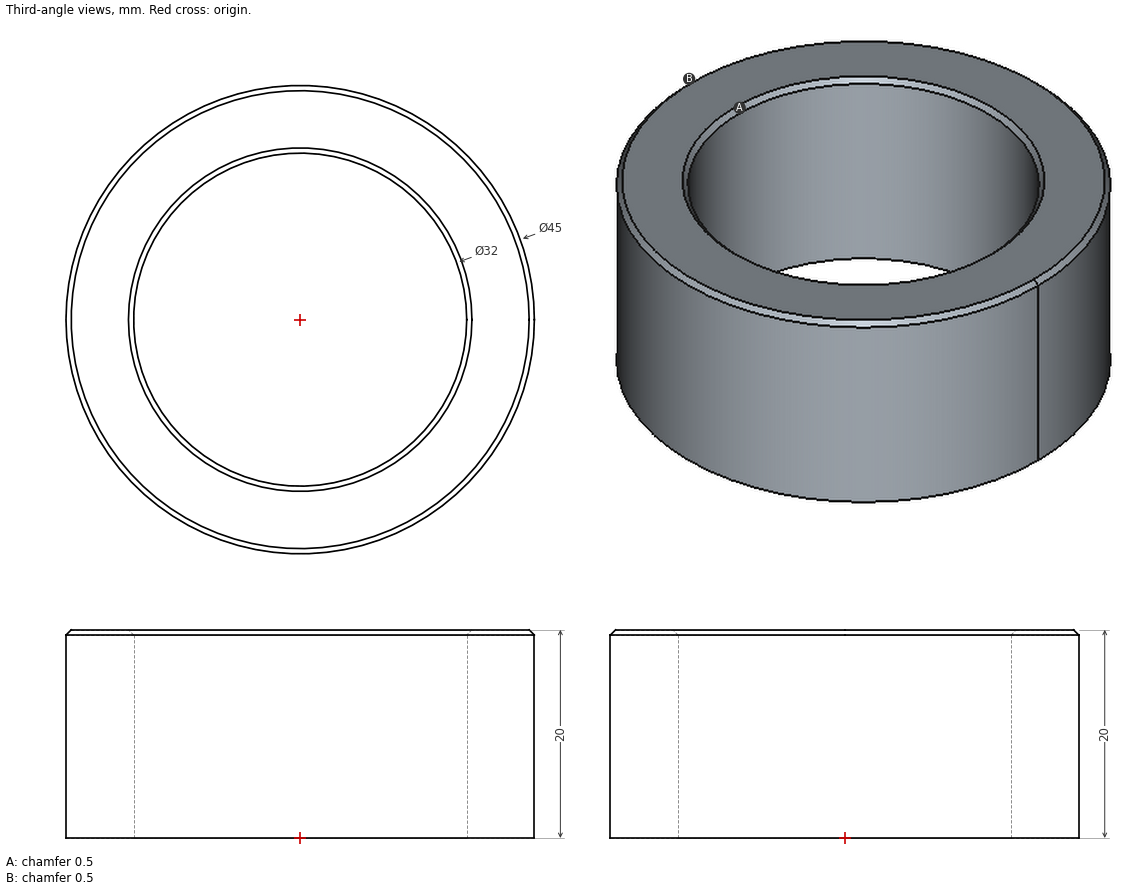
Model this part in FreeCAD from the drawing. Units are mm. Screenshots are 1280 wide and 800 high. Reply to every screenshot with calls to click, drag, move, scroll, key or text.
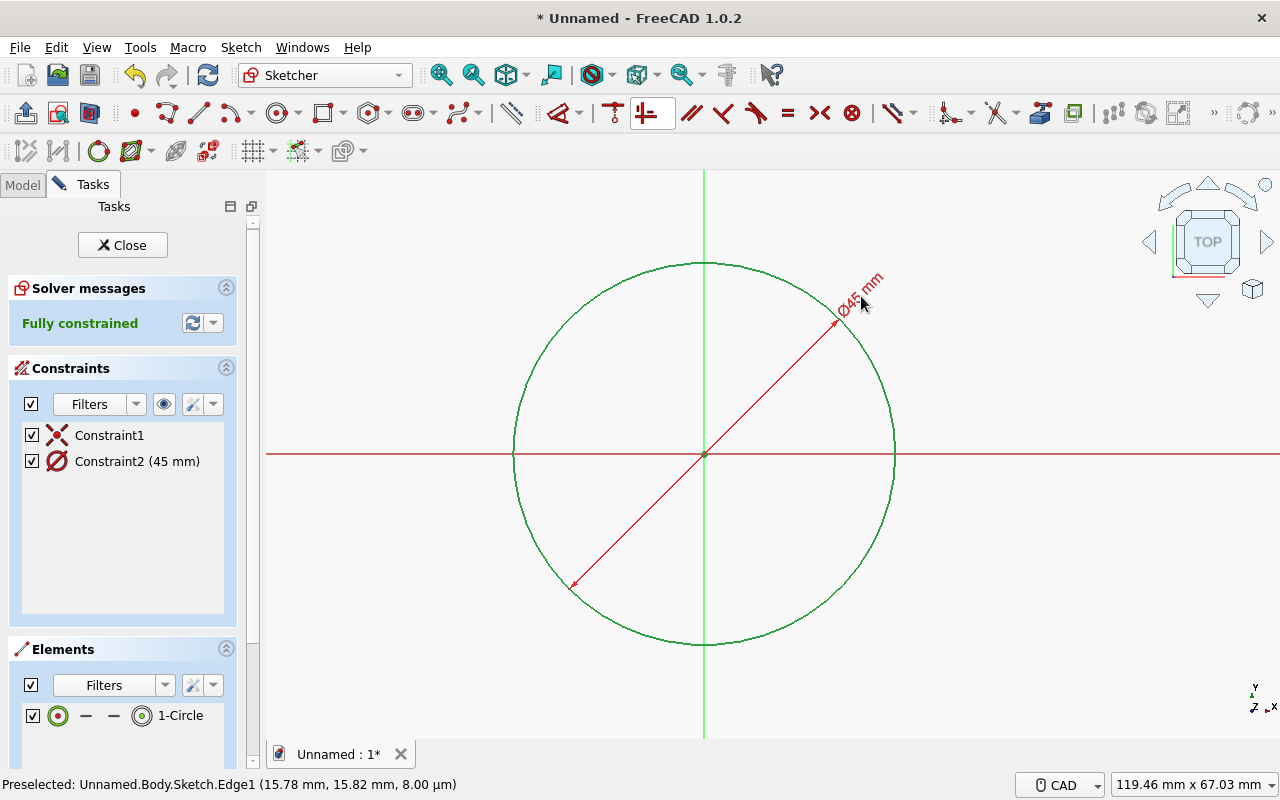
click(123, 245)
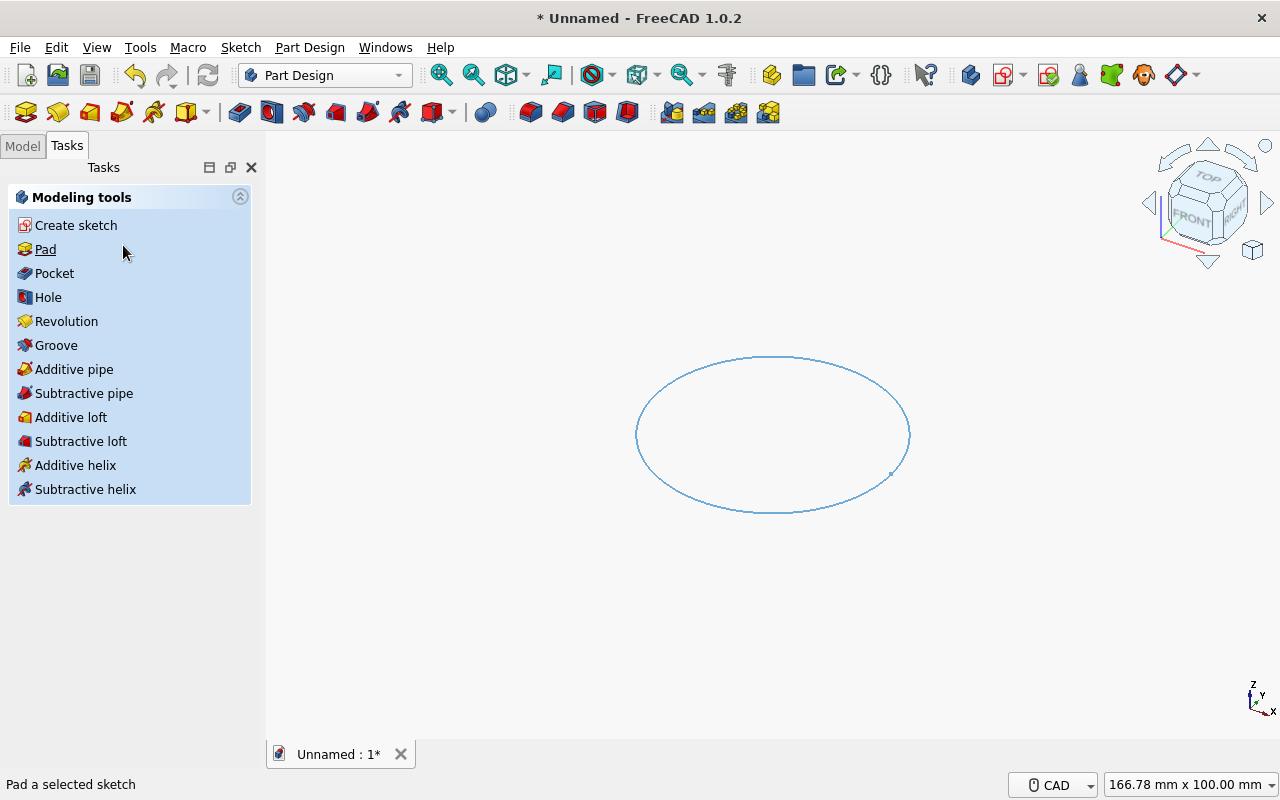
click(26, 112)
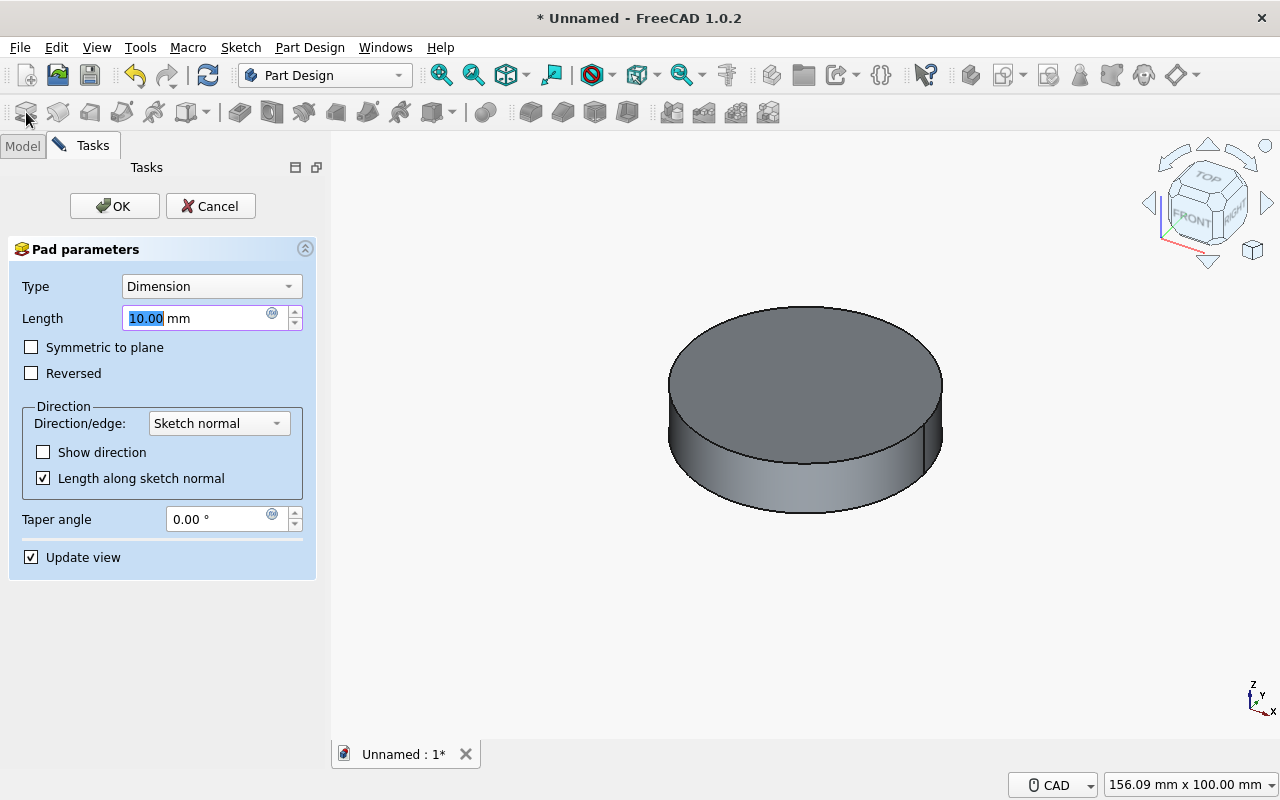
text(20)
key(Tab)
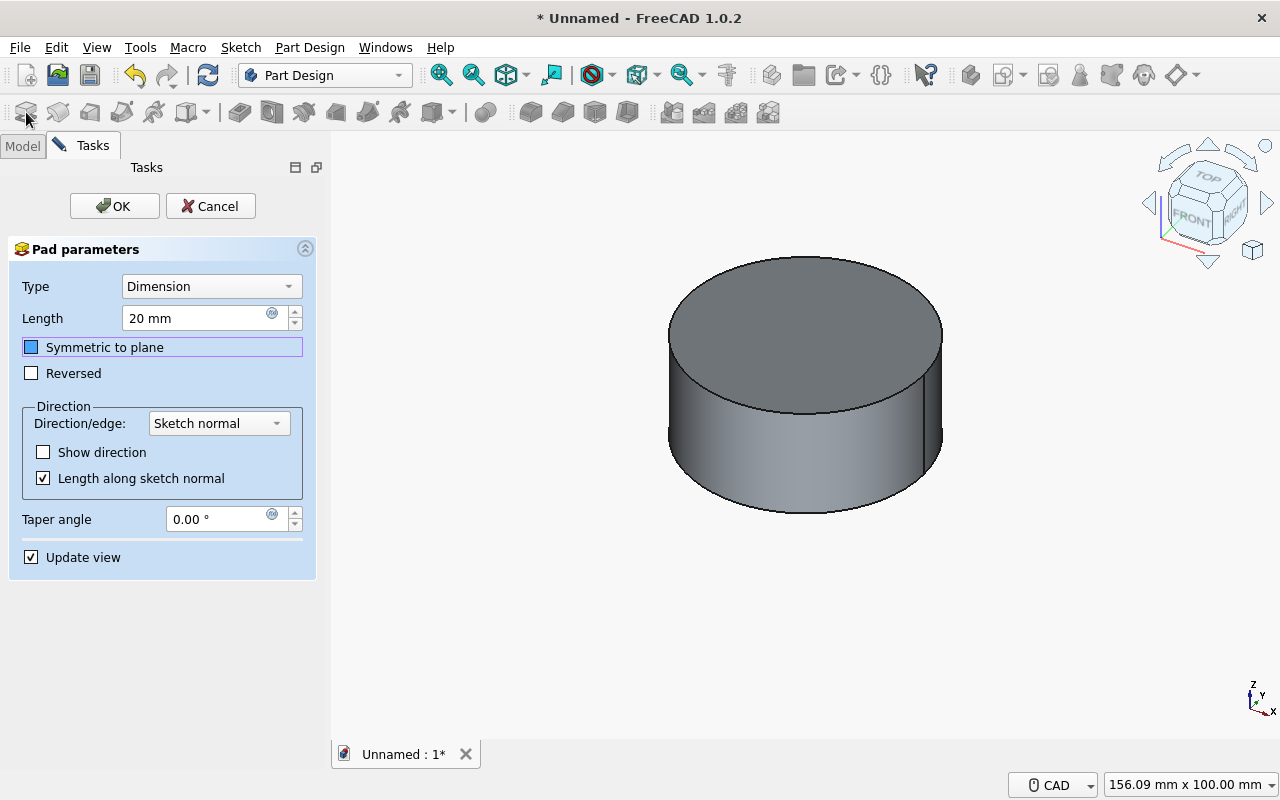
click(115, 206)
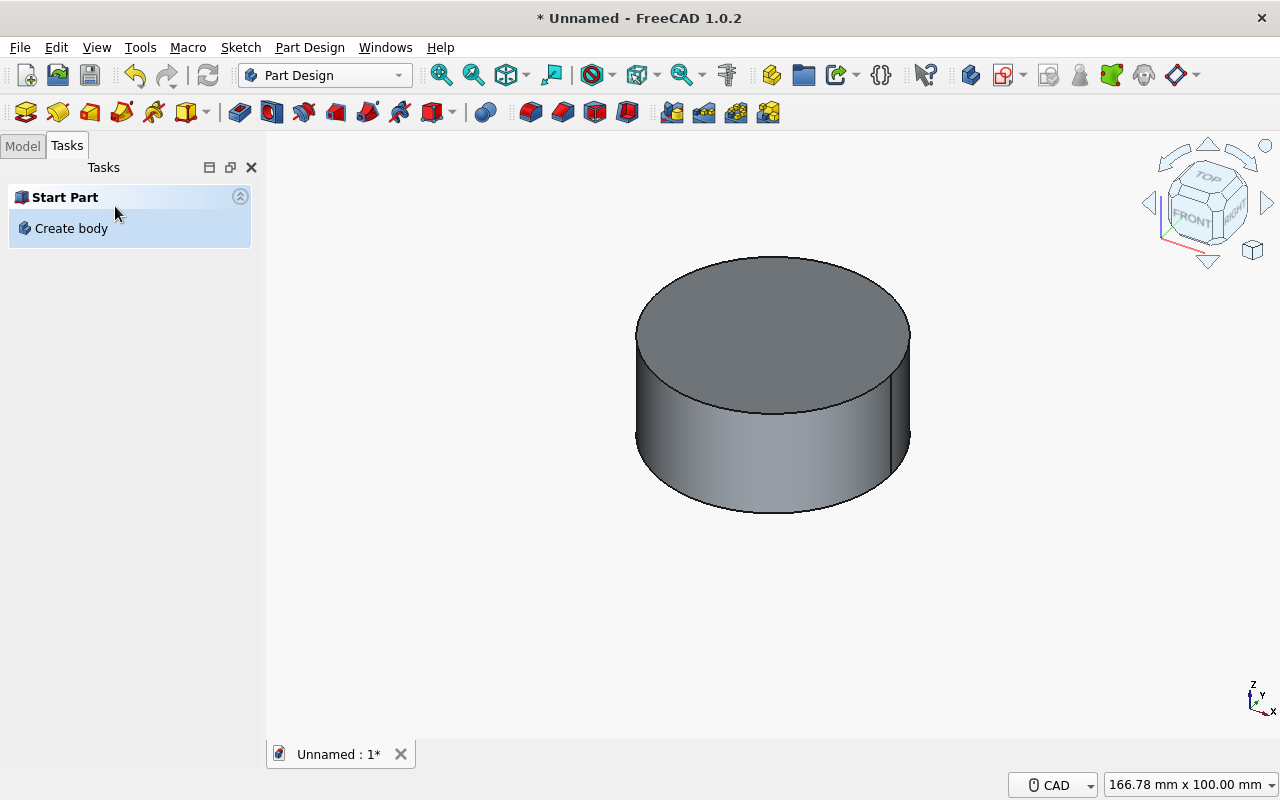
click(773, 334)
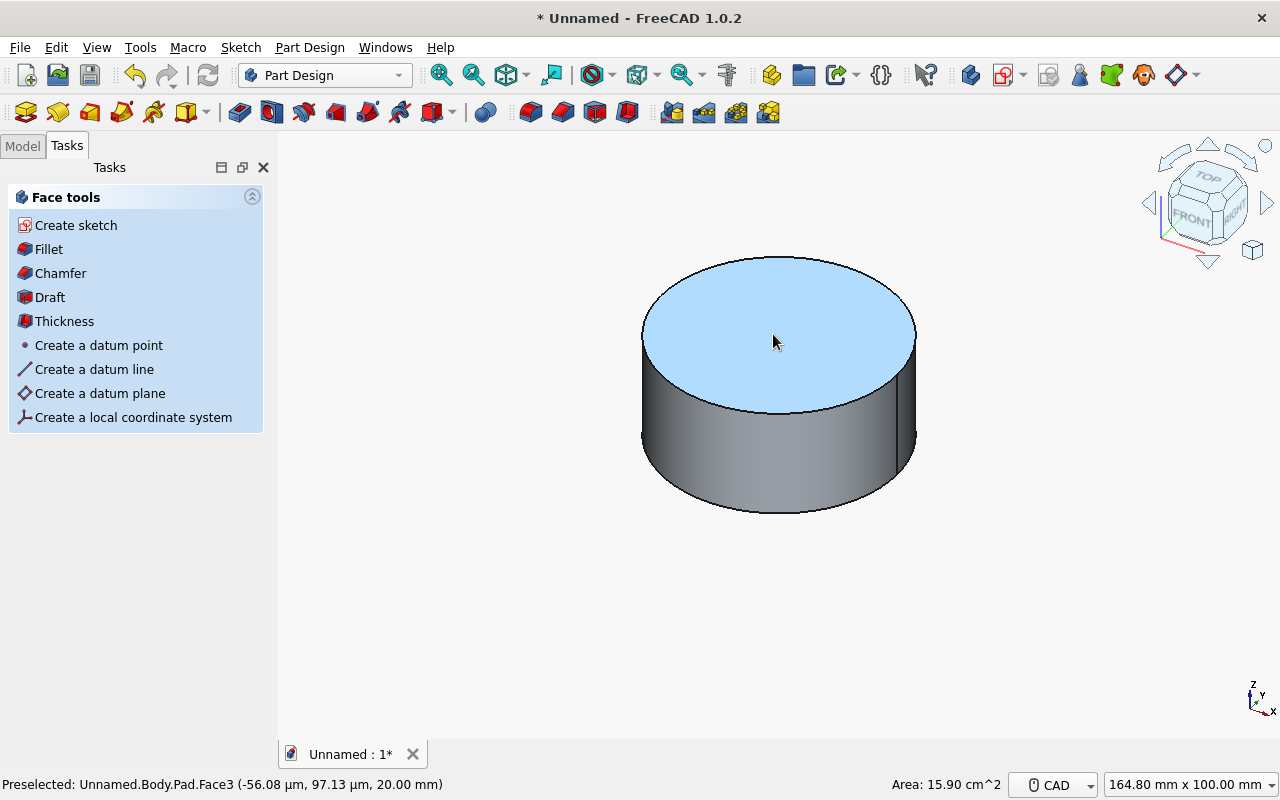
click(1004, 76)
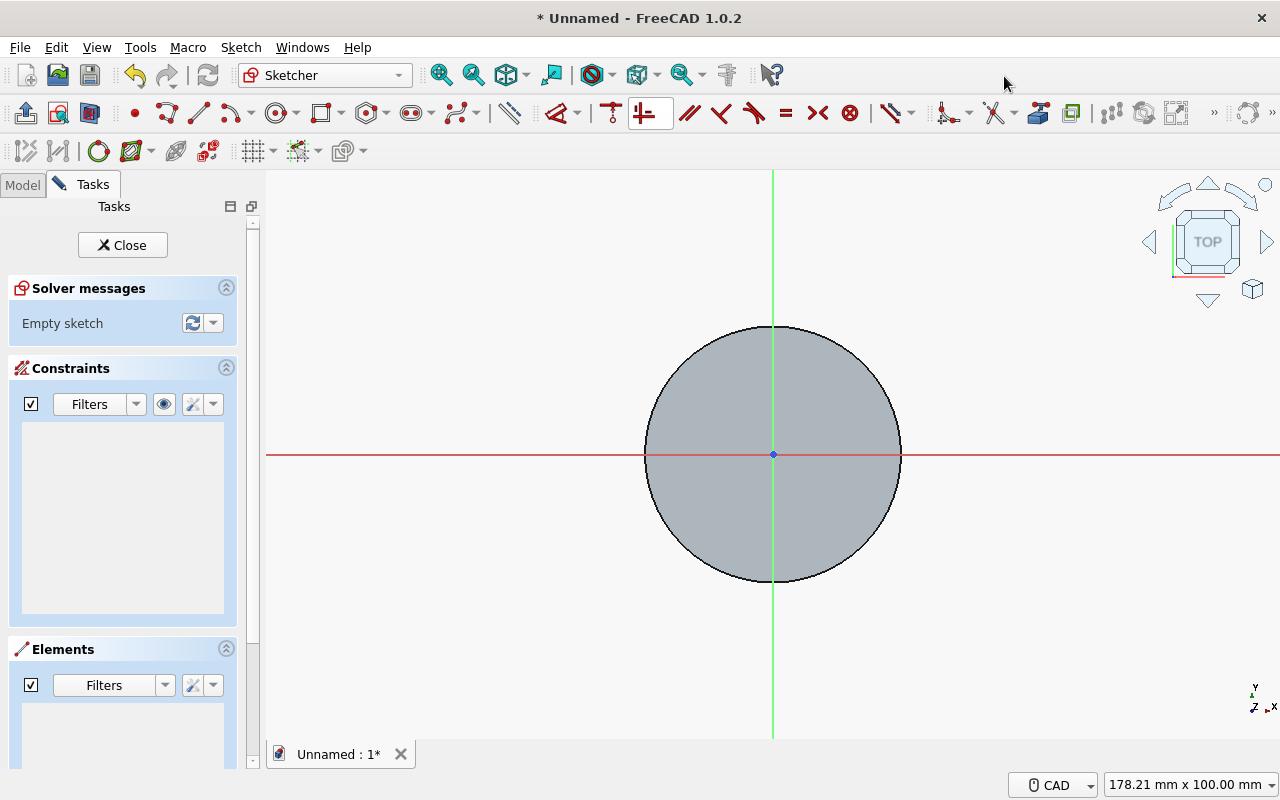
scroll(856, 454, up, 3)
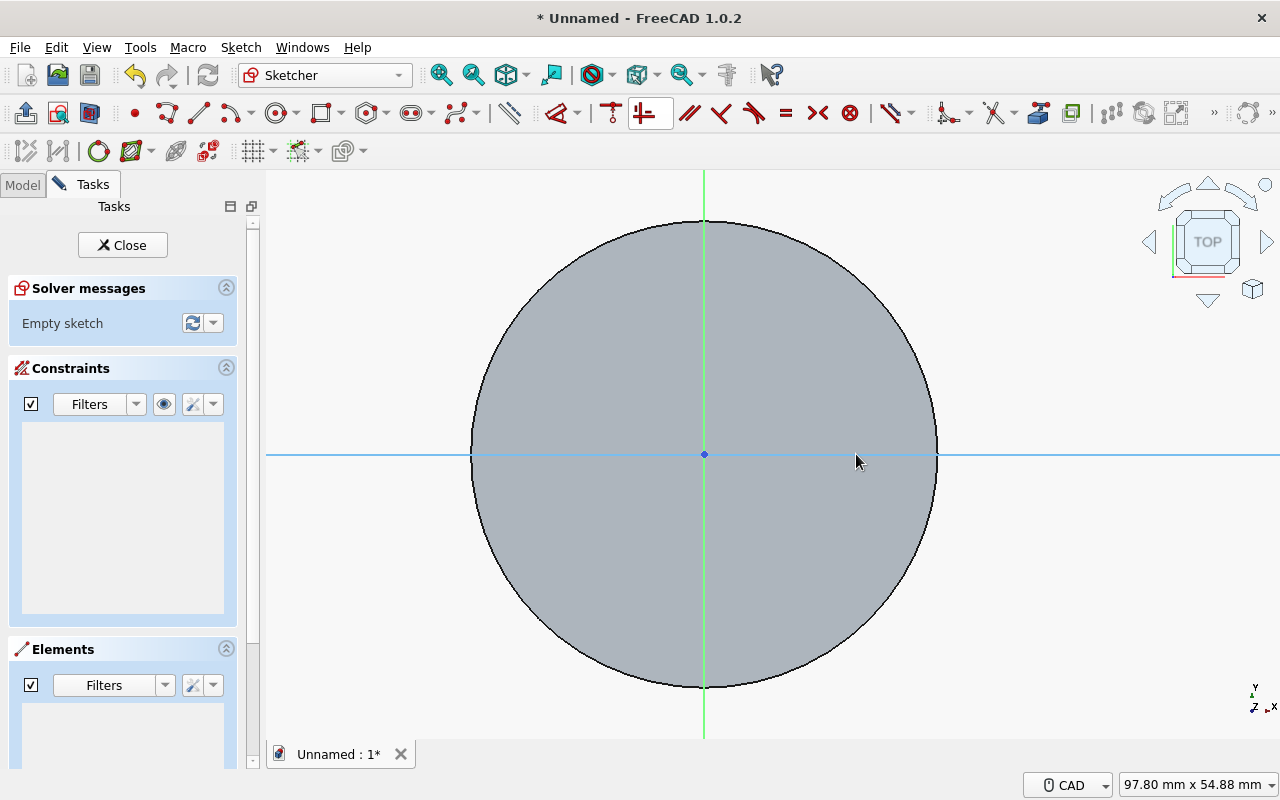
key(g)
key(c)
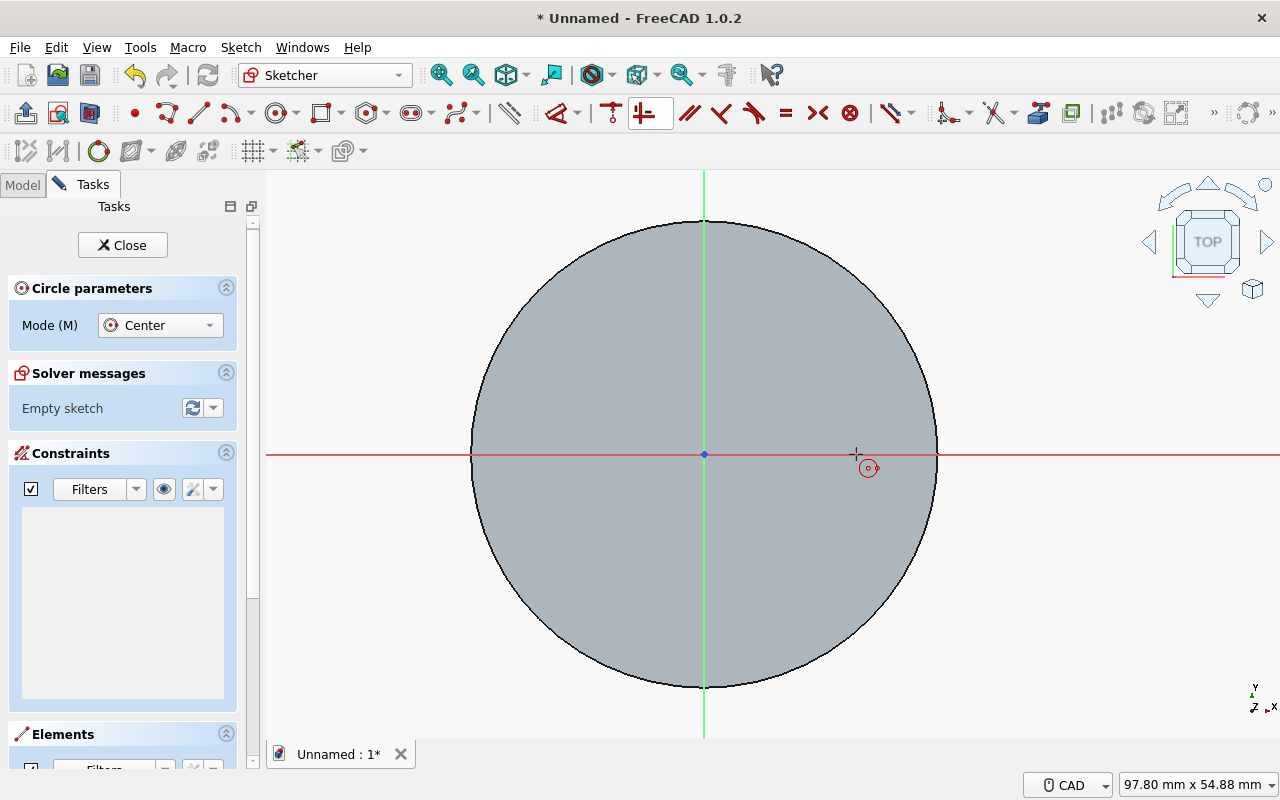
click(704, 454)
click(822, 337)
key(Escape)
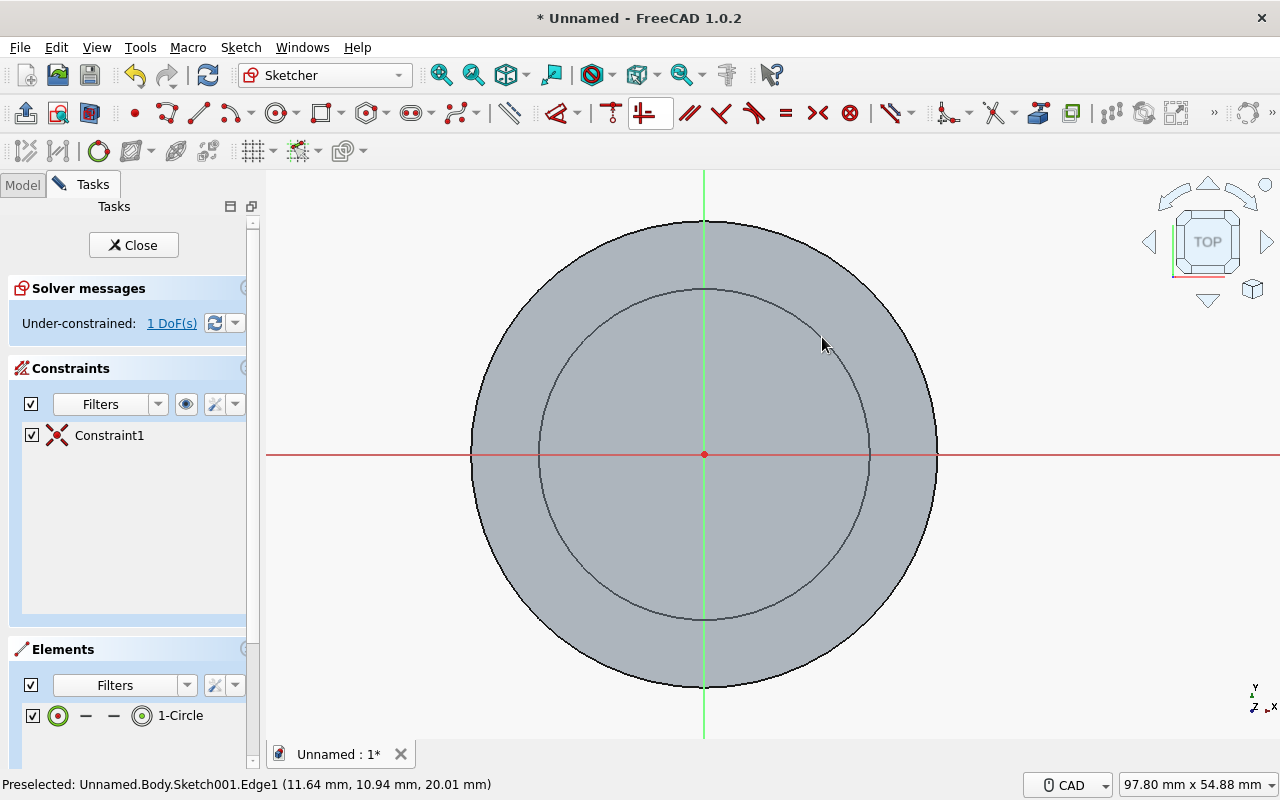
click(556, 114)